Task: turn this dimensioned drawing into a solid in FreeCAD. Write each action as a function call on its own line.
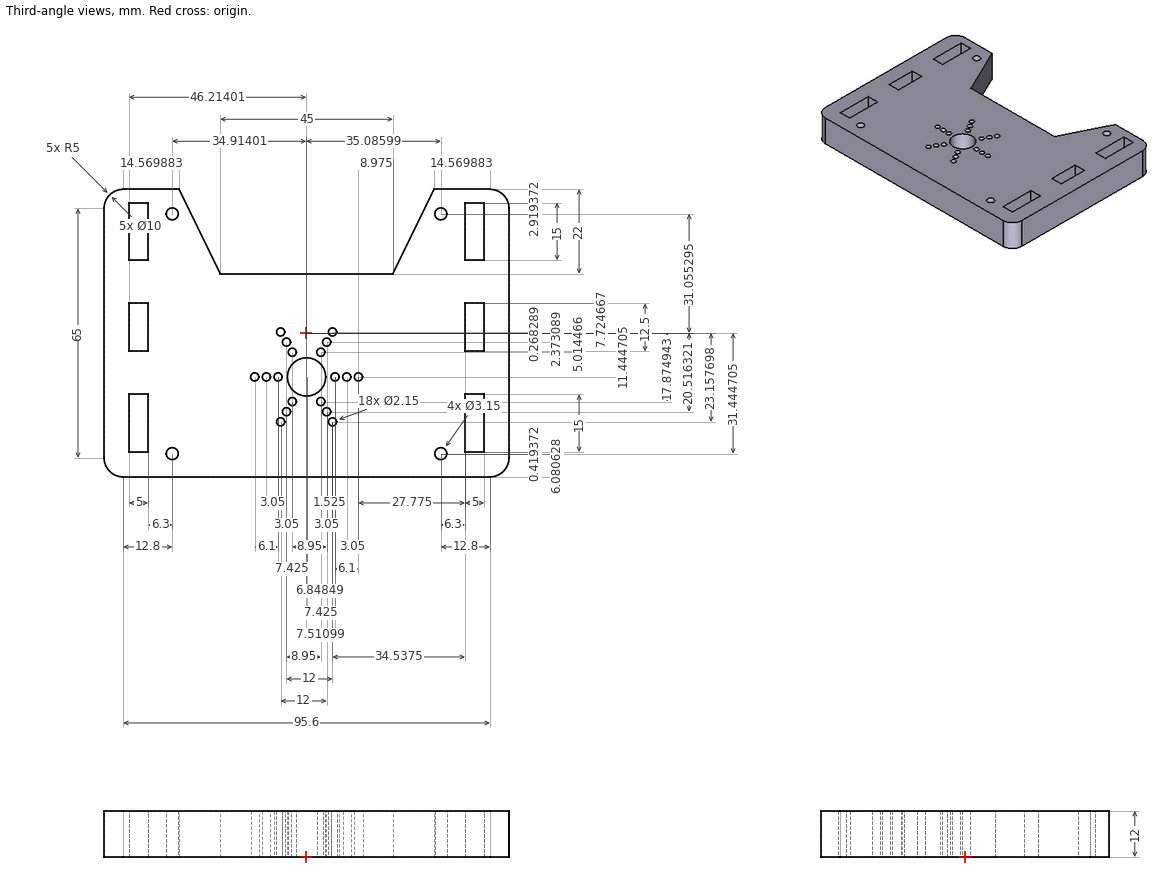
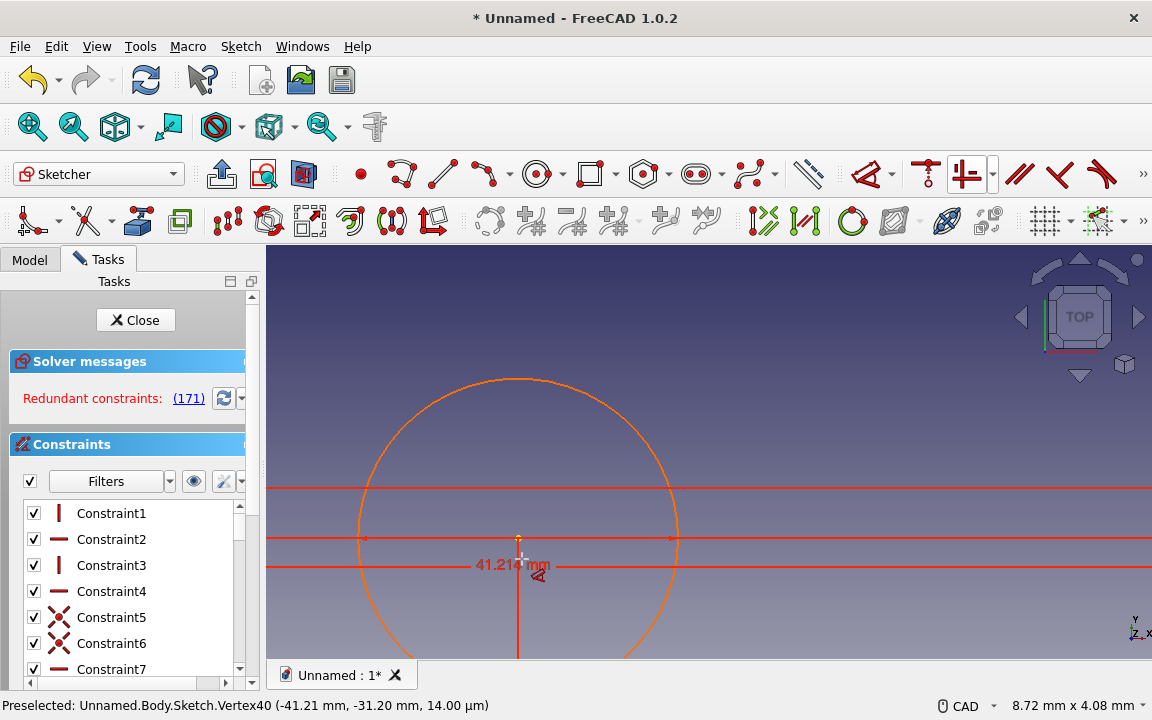
click(518, 538)
click(552, 526)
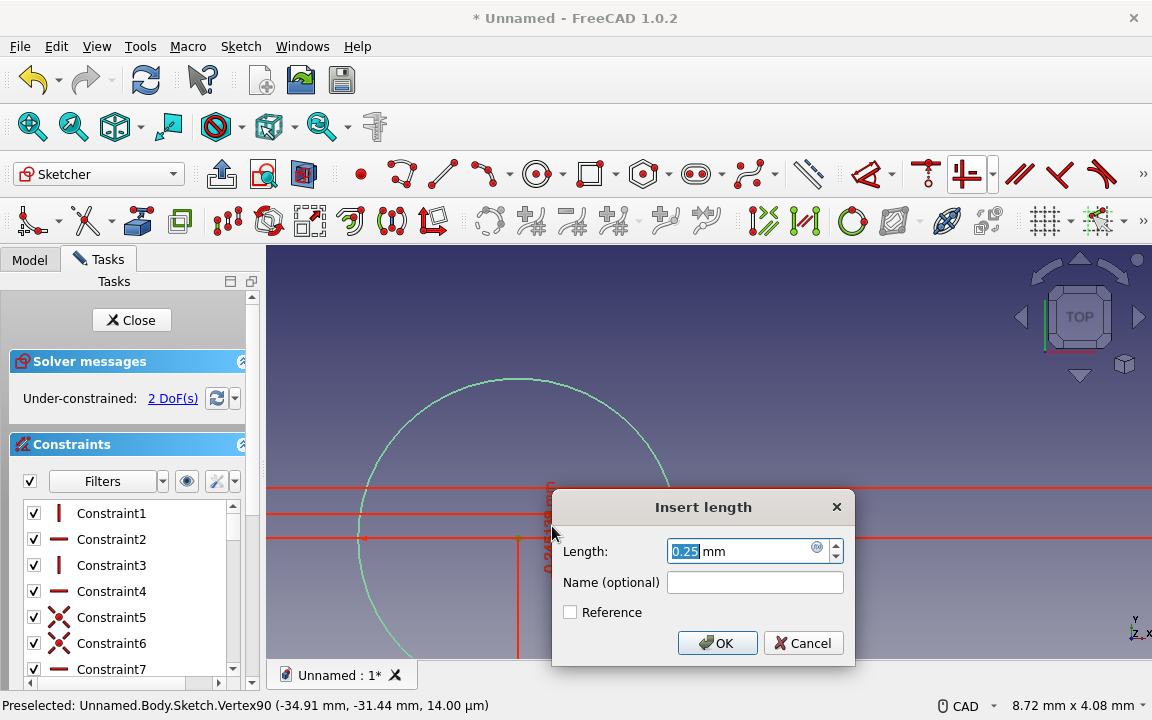
text(0.419372)
key(Return)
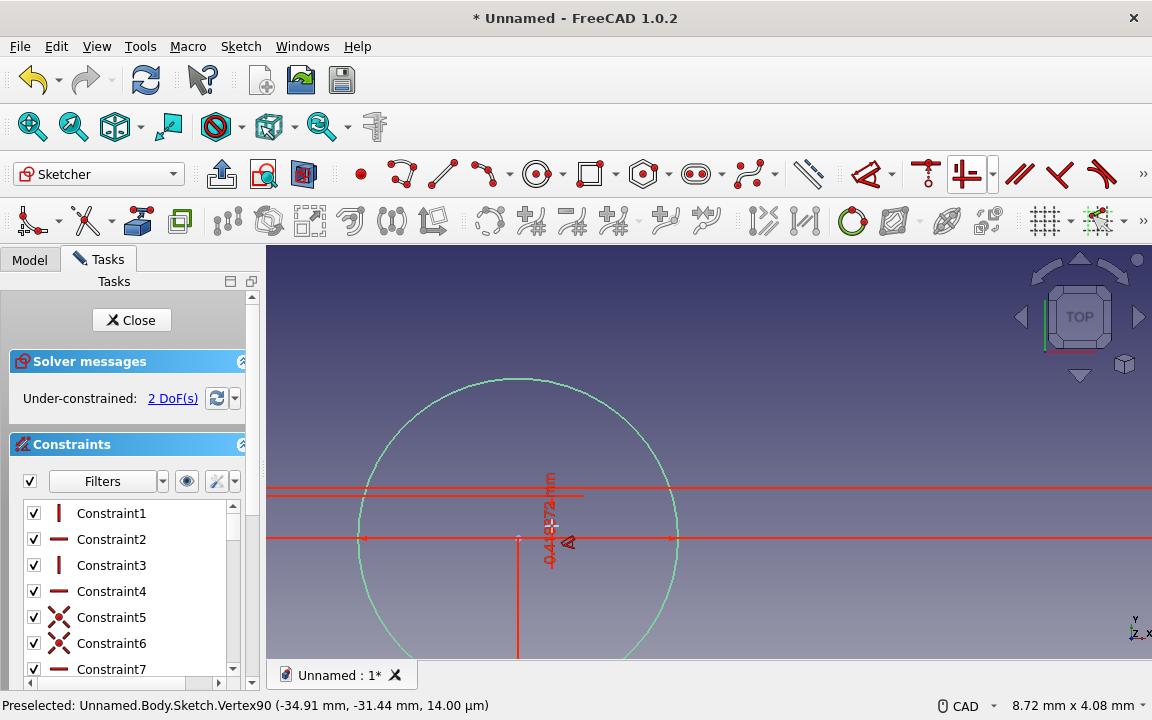
scroll(522, 559, down, 17)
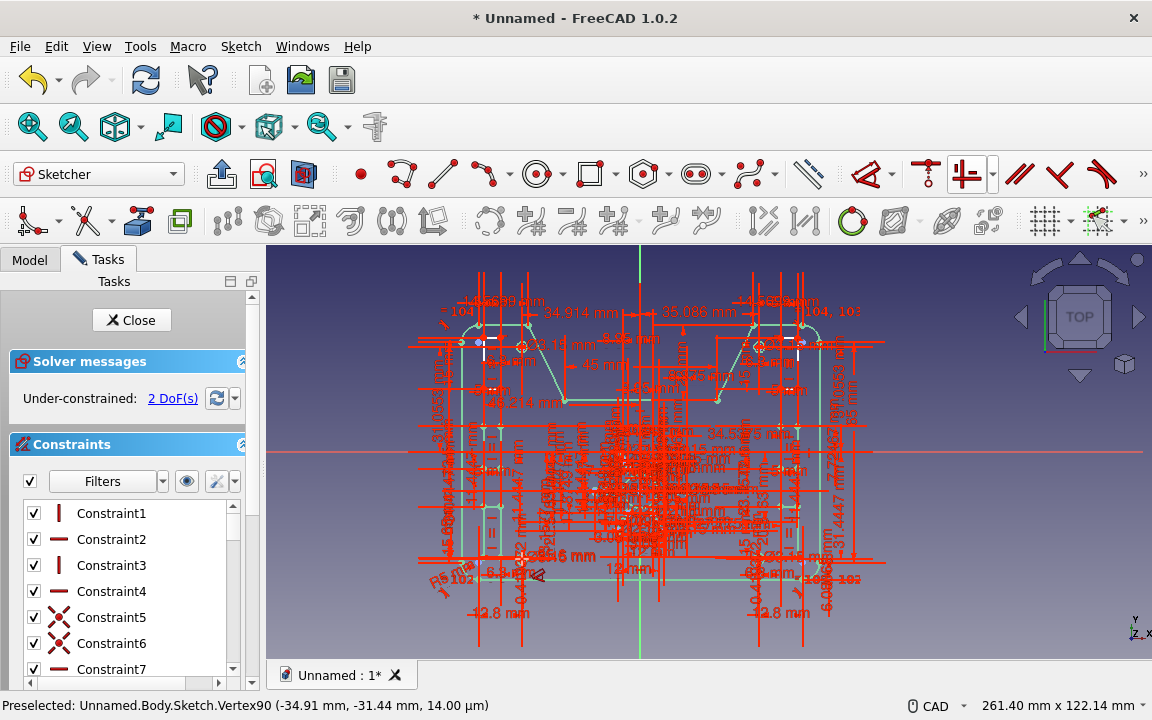
scroll(781, 338, up, 7)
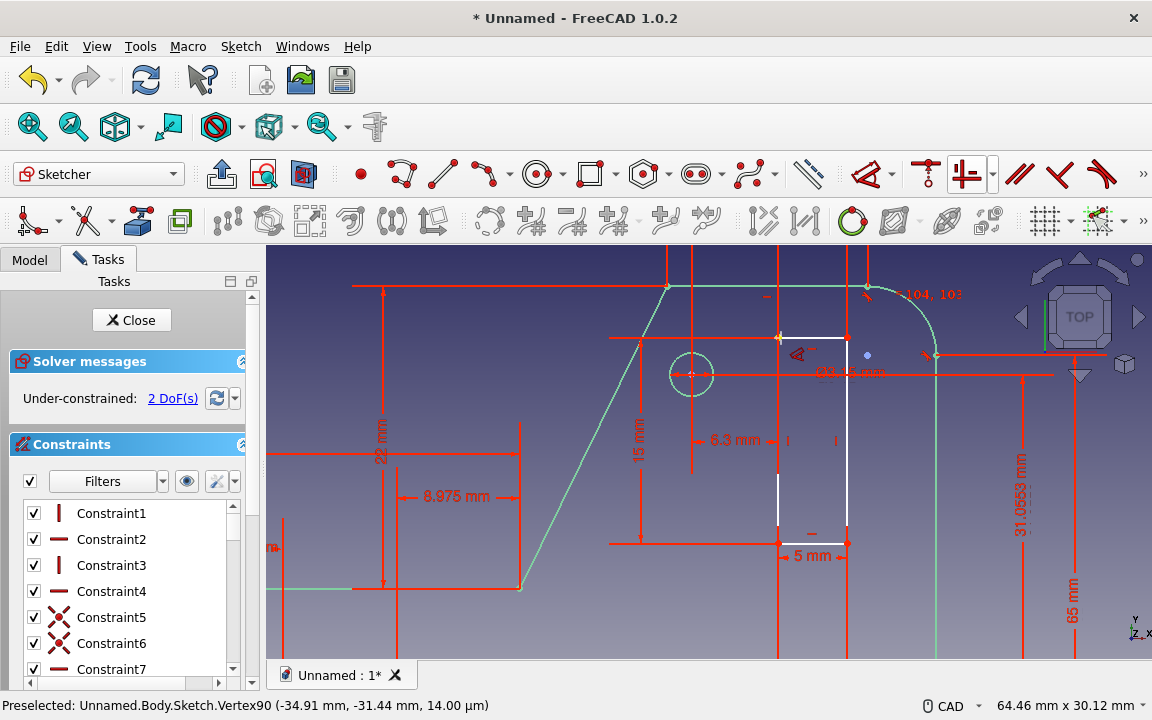
click(778, 338)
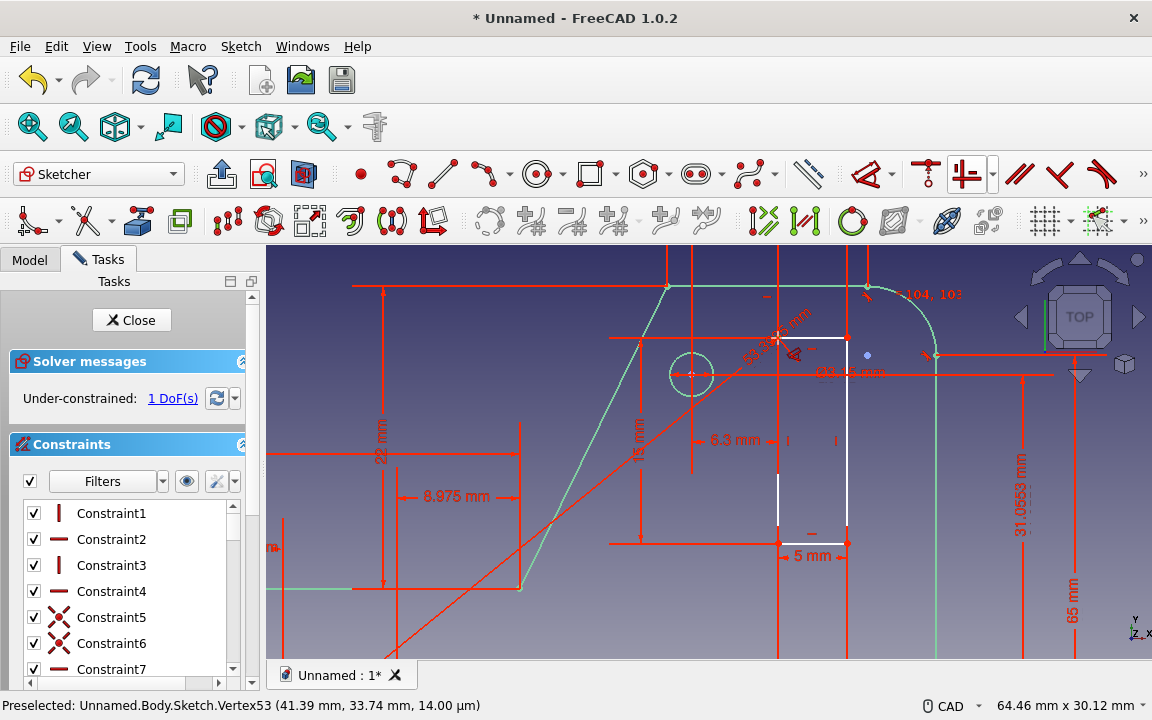
click(692, 375)
click(812, 356)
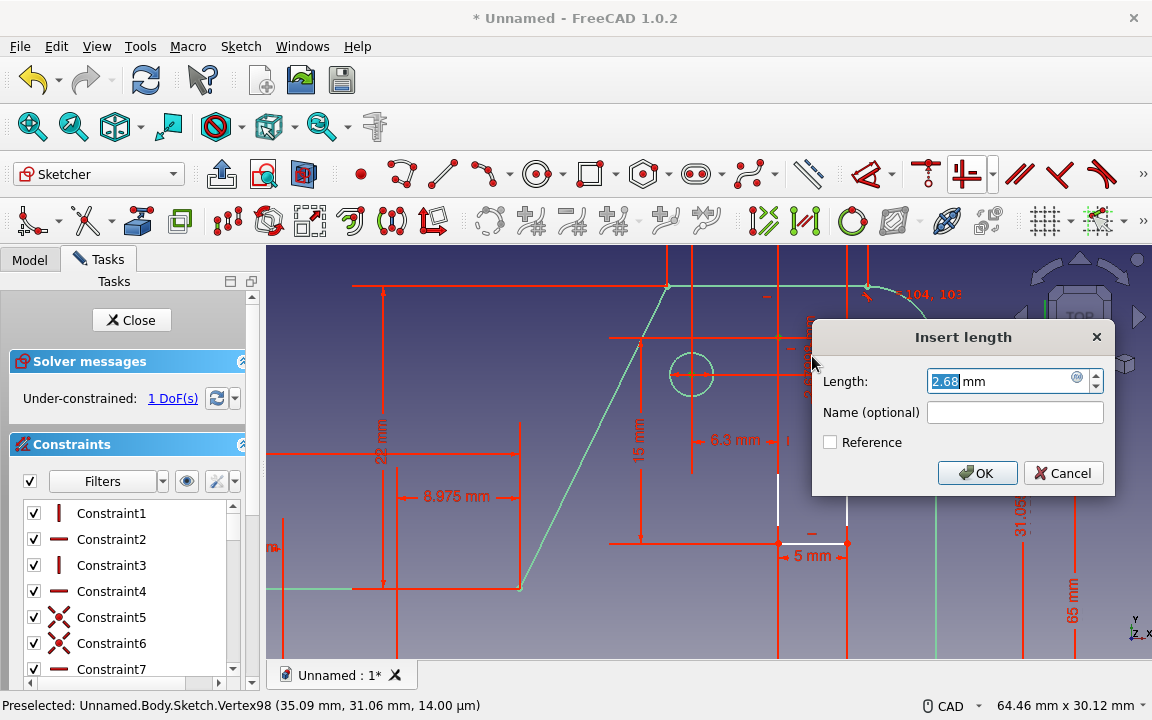
text(2.919372)
key(Return)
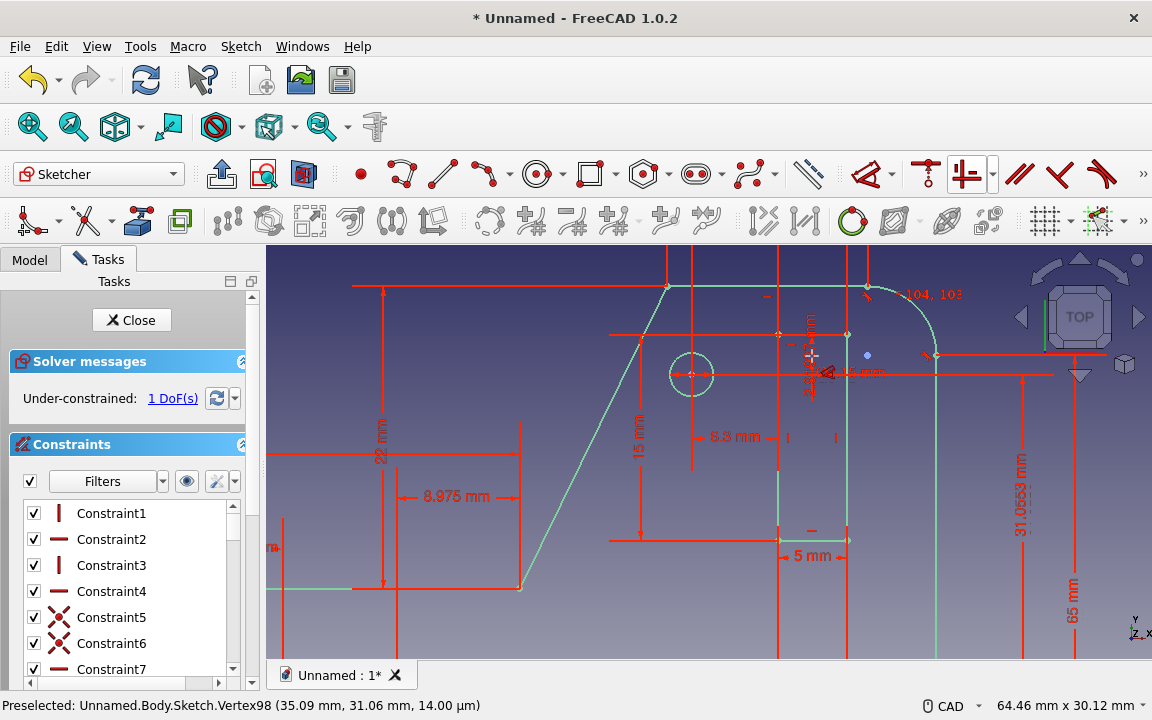
scroll(781, 337, down, 7)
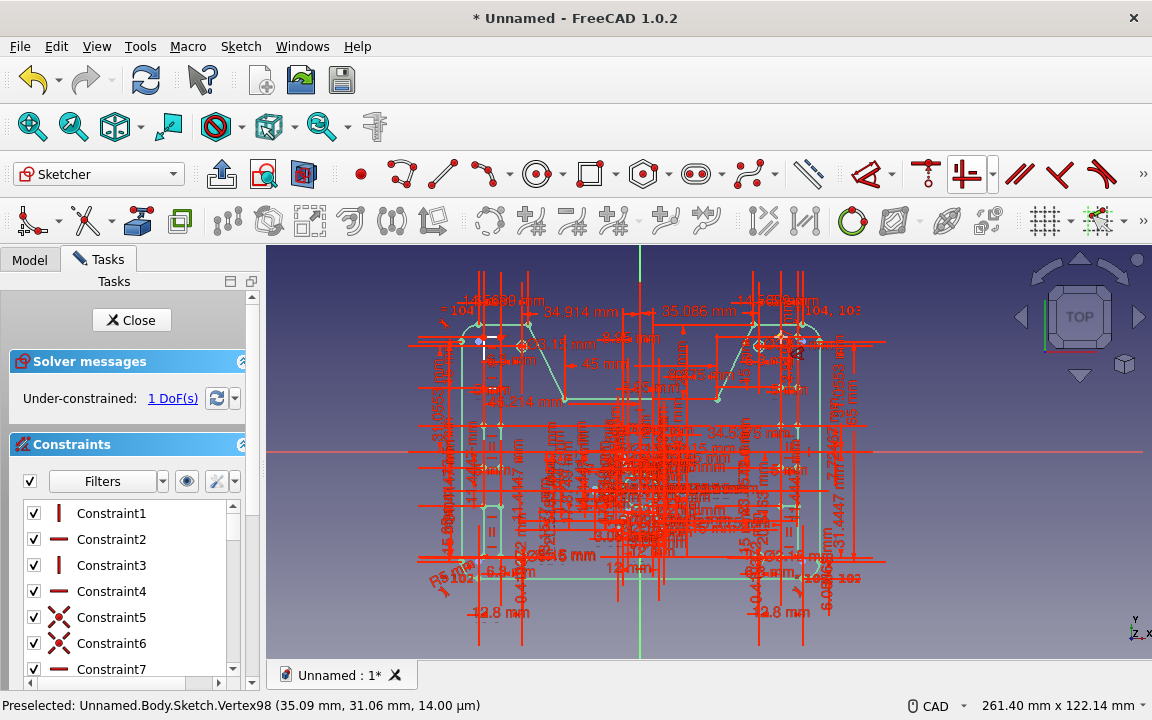
scroll(501, 337, up, 7)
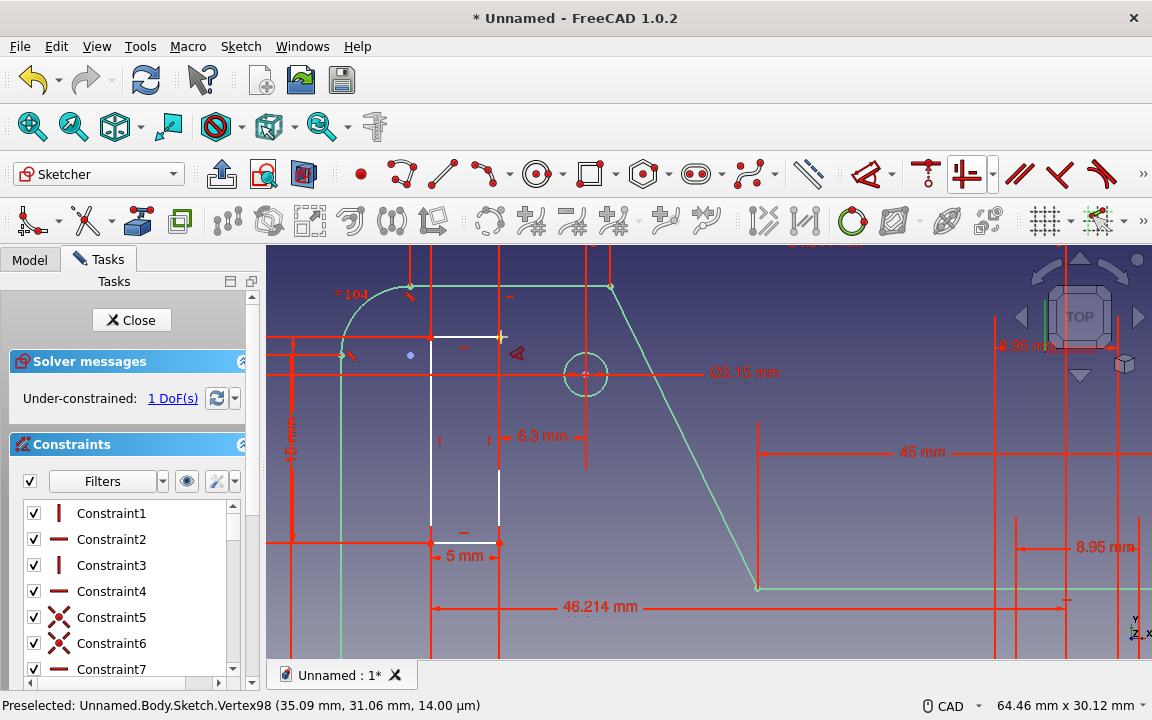
click(499, 337)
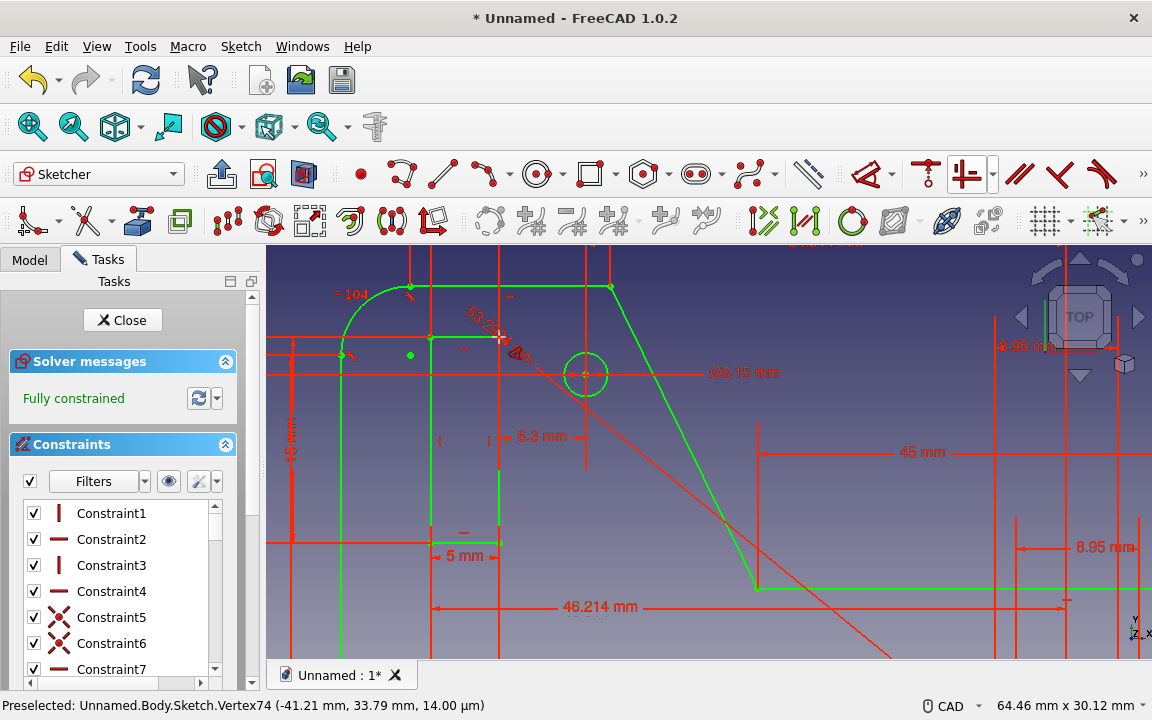
click(586, 375)
click(465, 356)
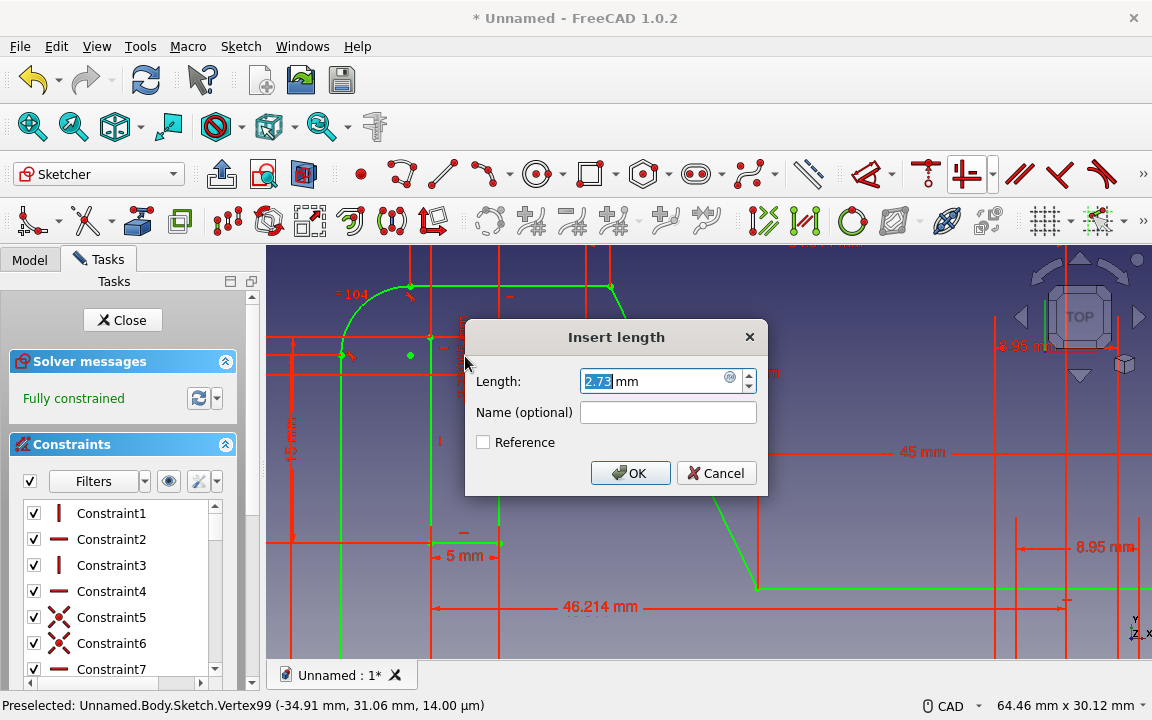
text(2.919372)
key(Return)
key(Escape)